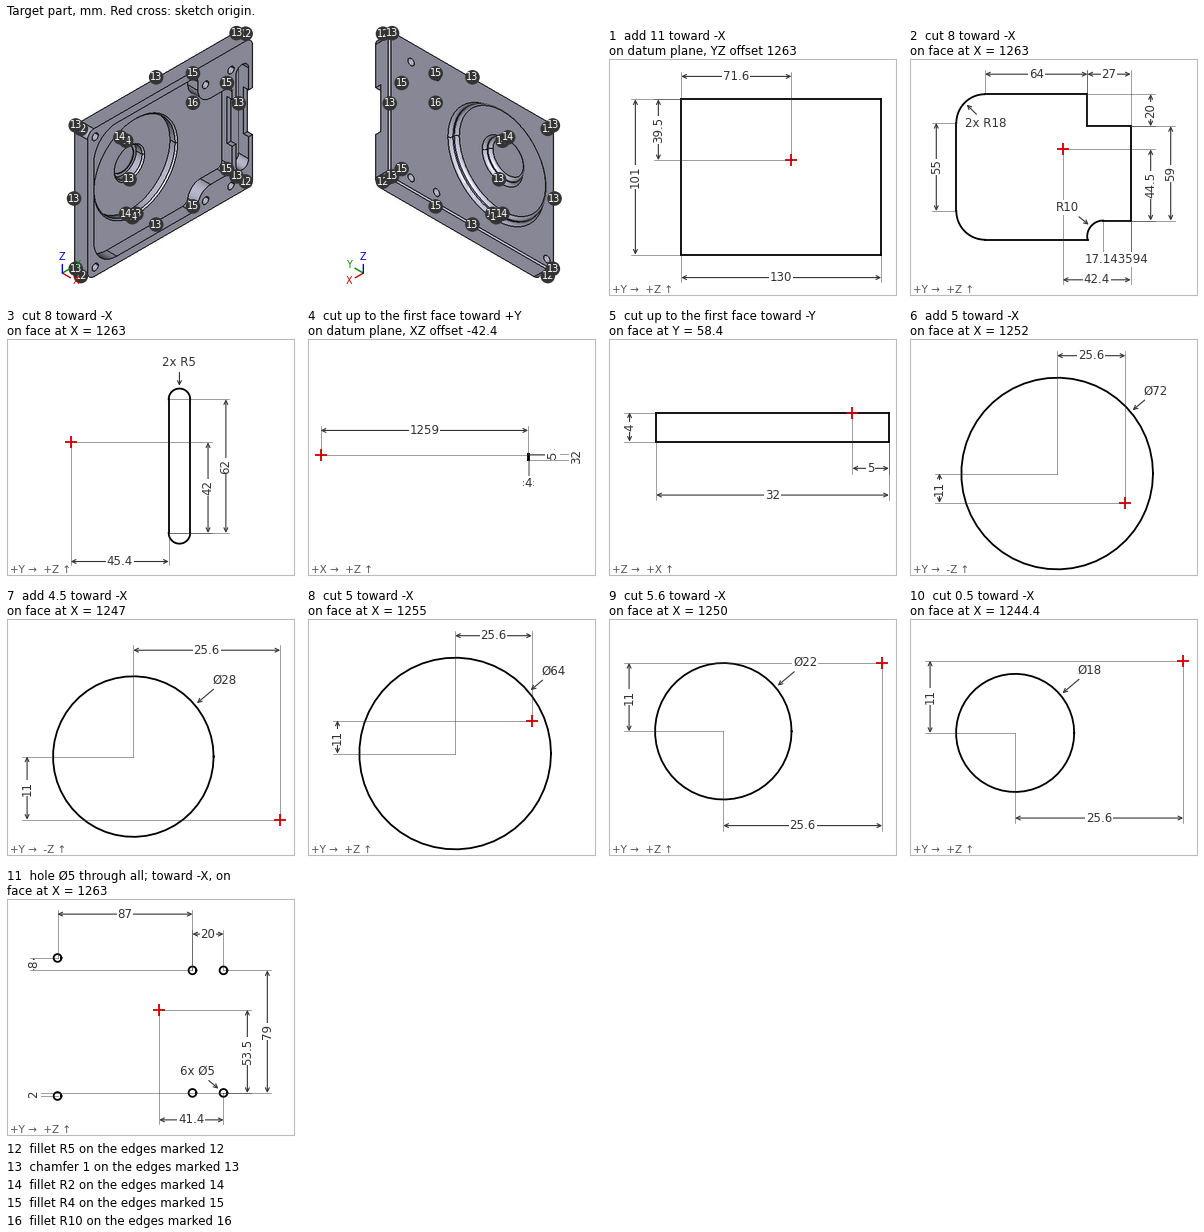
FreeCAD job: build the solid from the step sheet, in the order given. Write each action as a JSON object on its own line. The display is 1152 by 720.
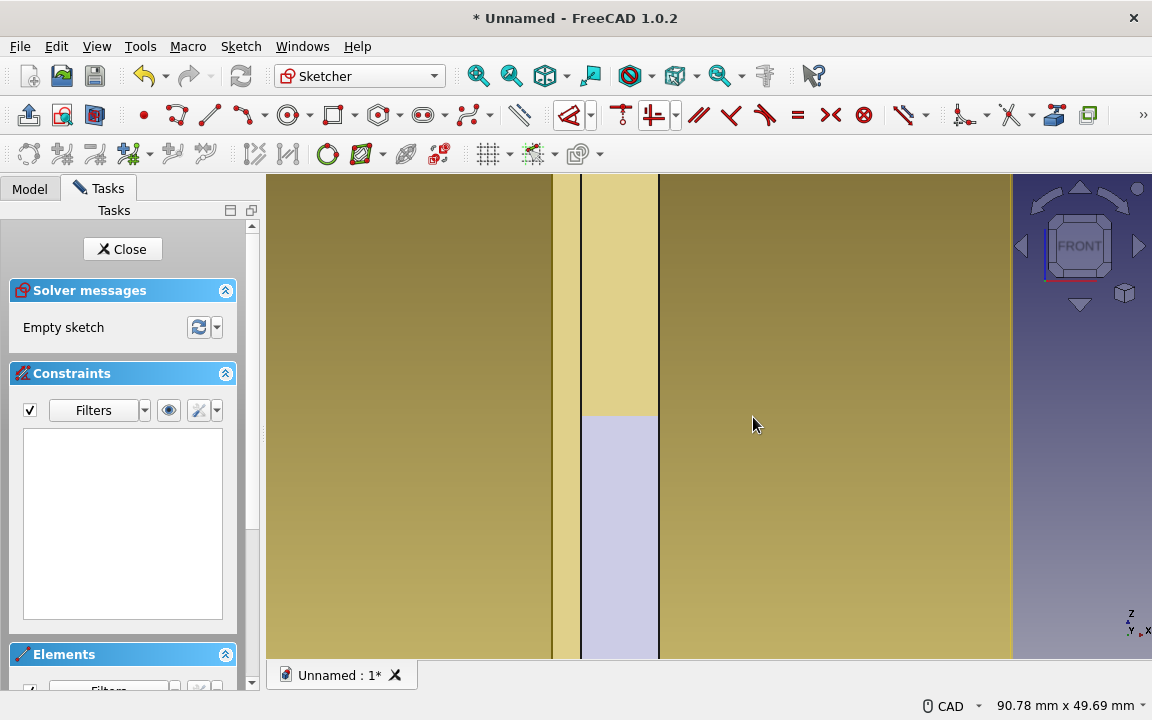
{"action": "left_click", "coordinate": [332, 116]}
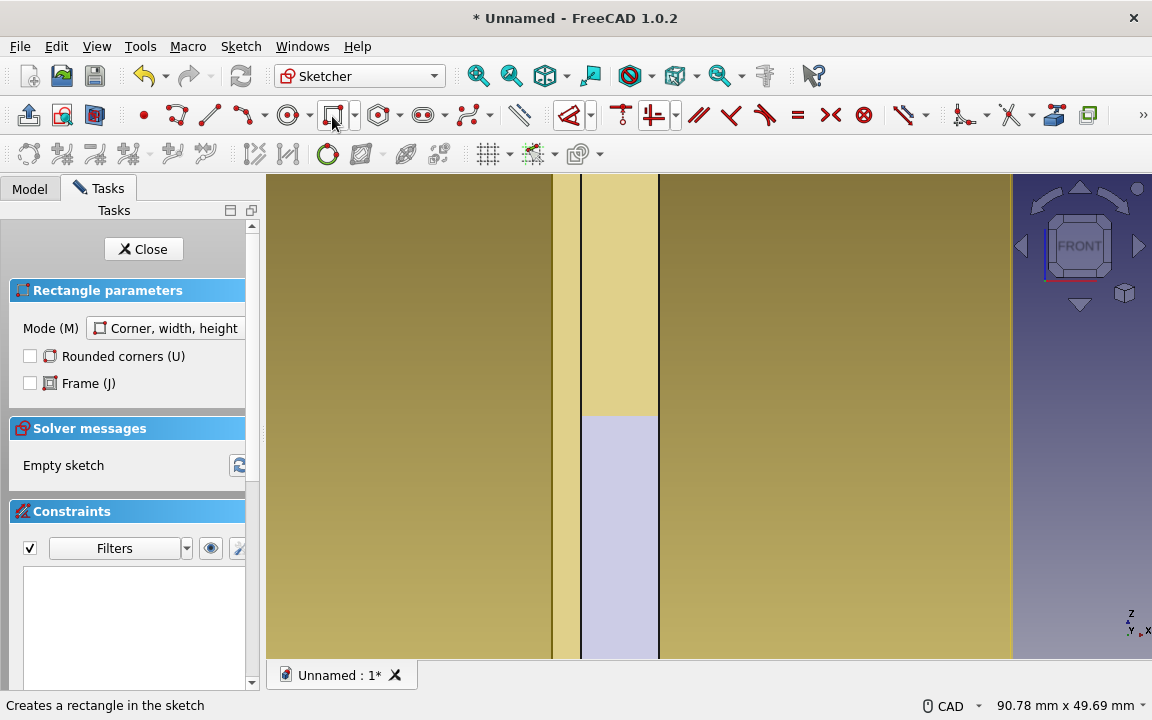
{"action": "left_click", "coordinate": [620, 258]}
{"action": "left_click", "coordinate": [659, 570]}
{"action": "key", "text": "Escape"}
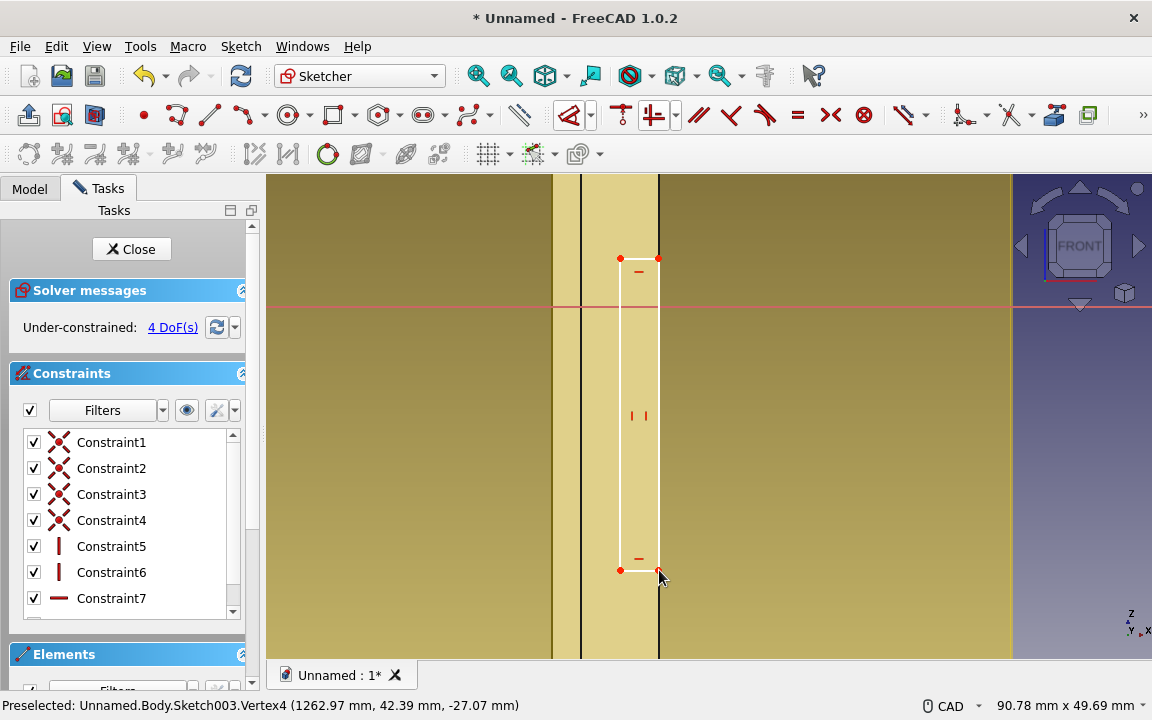
{"action": "left_click", "coordinate": [632, 571]}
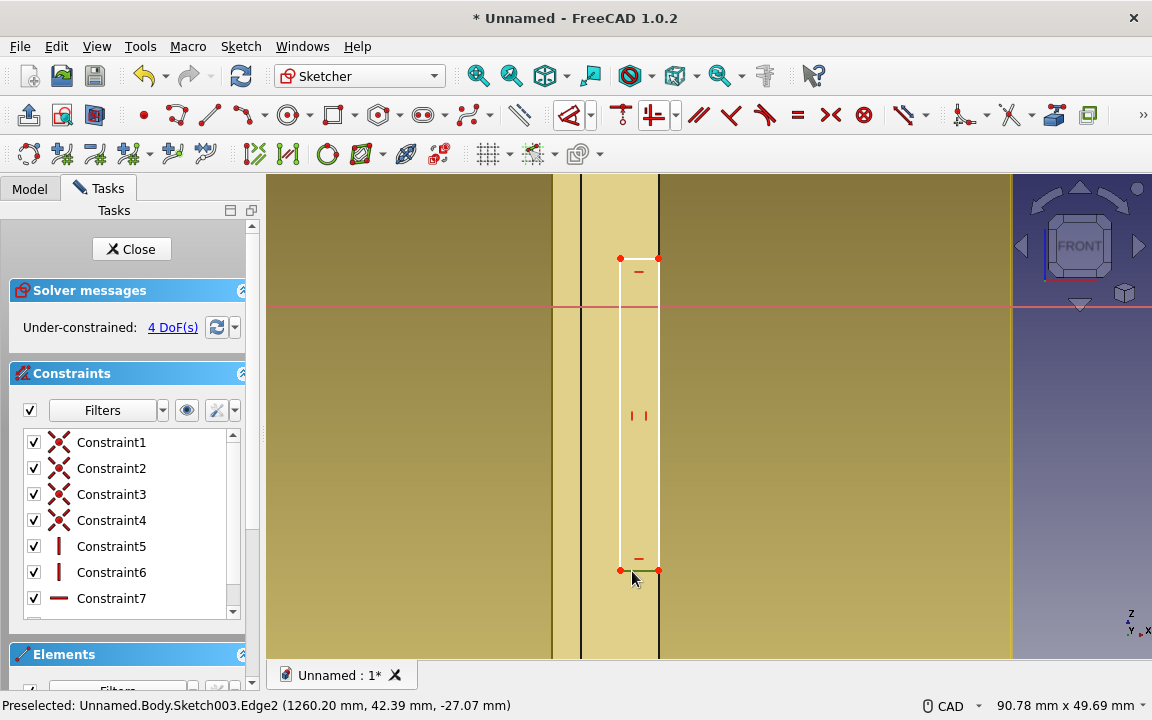
{"action": "left_click", "coordinate": [590, 116]}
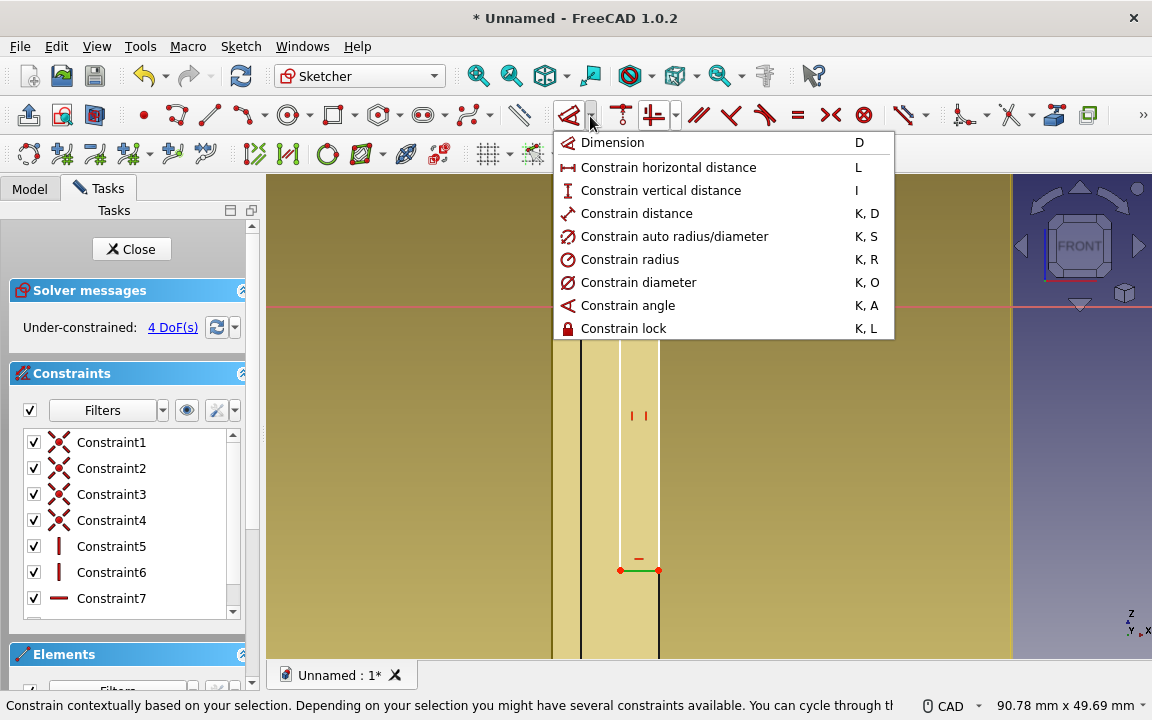
{"action": "left_click", "coordinate": [724, 168]}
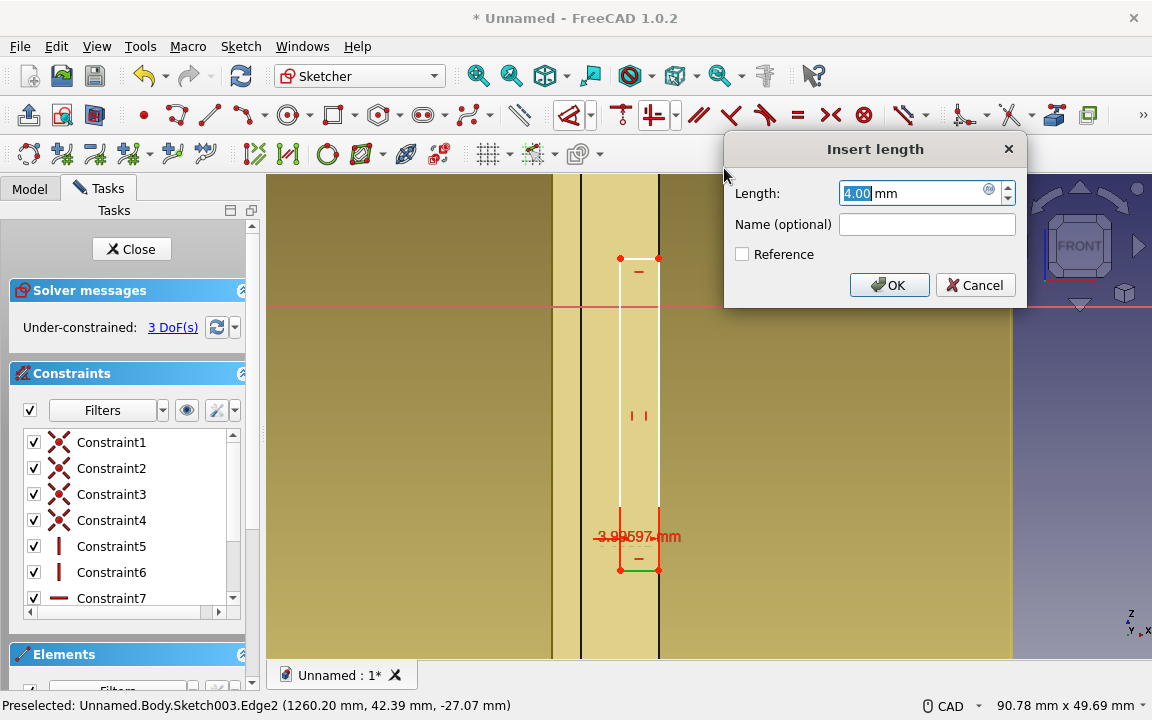
{"action": "type", "text": "4"}
{"action": "key", "text": "Return"}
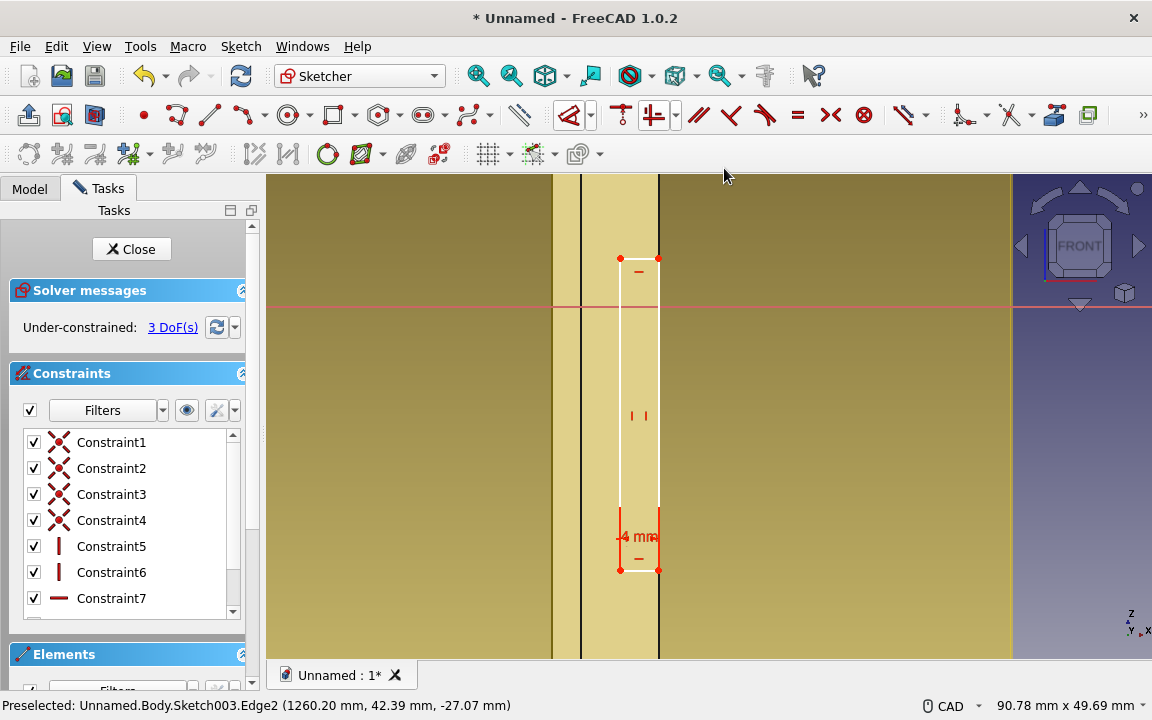
{"action": "left_click", "coordinate": [620, 353]}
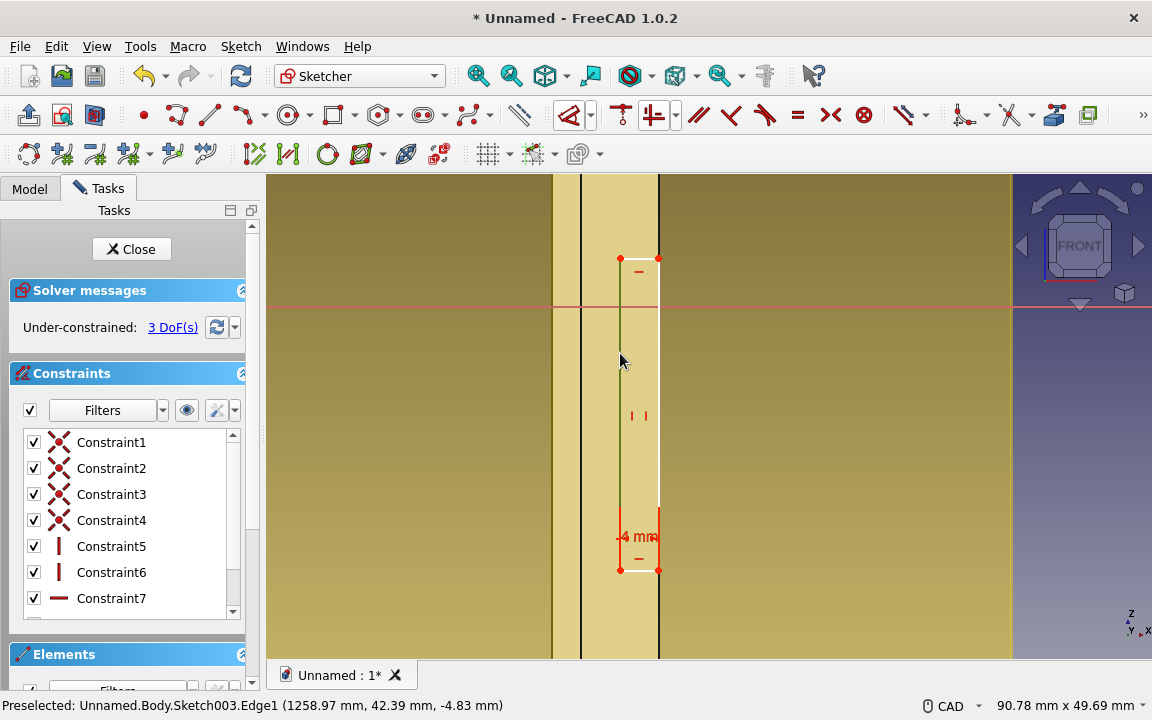
{"action": "left_click", "coordinate": [590, 116]}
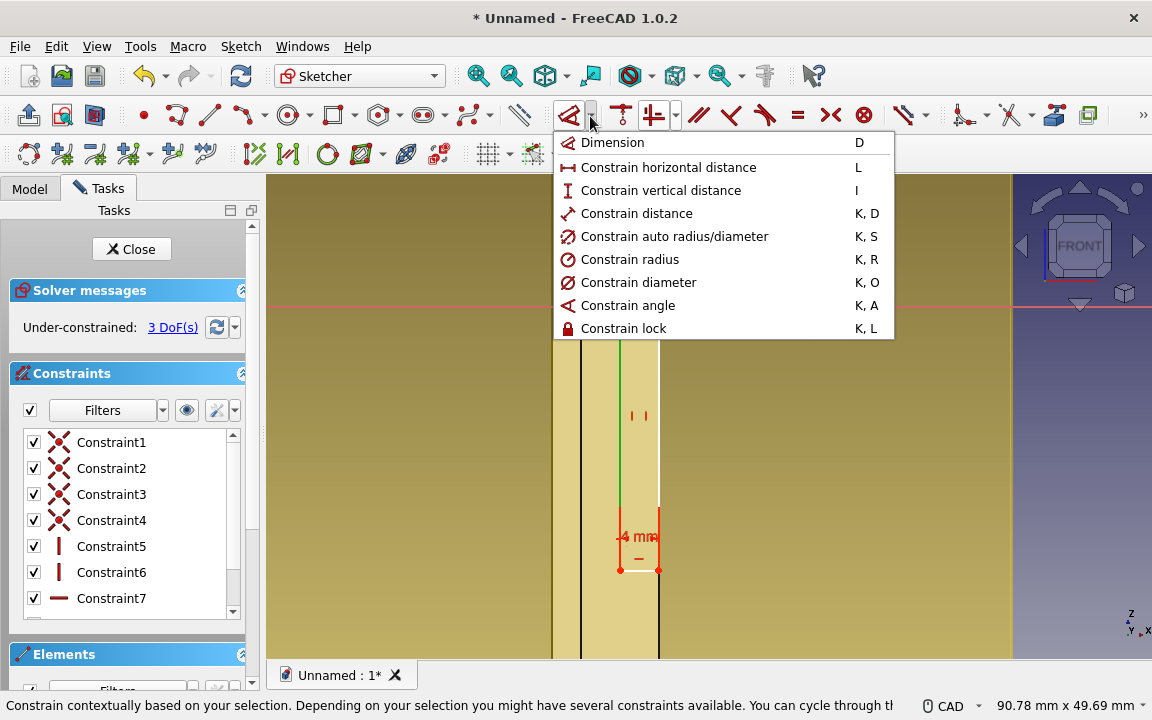
{"action": "left_click", "coordinate": [724, 190]}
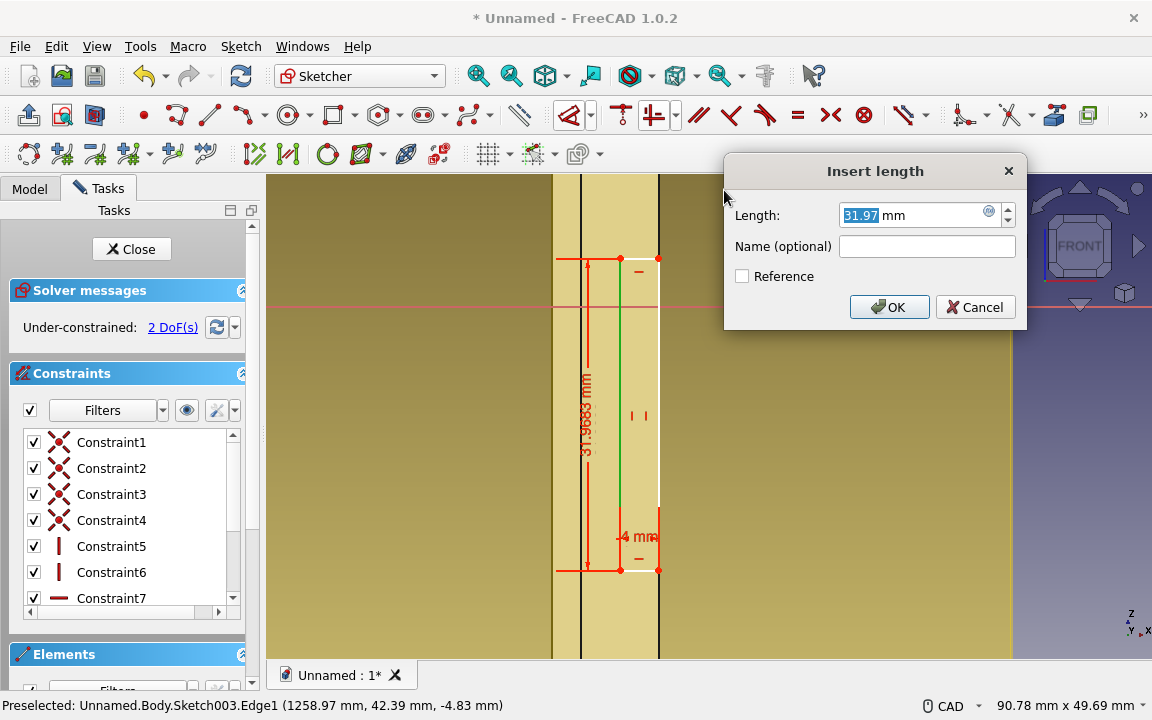
{"action": "type", "text": "32"}
{"action": "key", "text": "Return"}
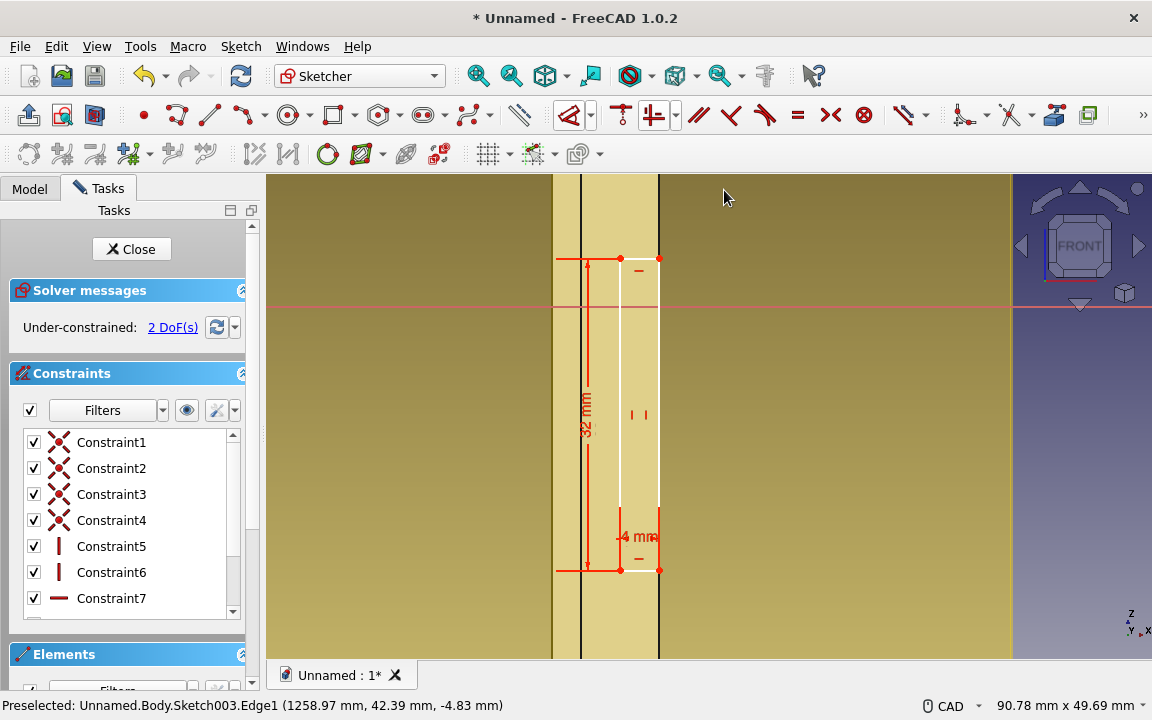
{"action": "left_click", "coordinate": [620, 259]}